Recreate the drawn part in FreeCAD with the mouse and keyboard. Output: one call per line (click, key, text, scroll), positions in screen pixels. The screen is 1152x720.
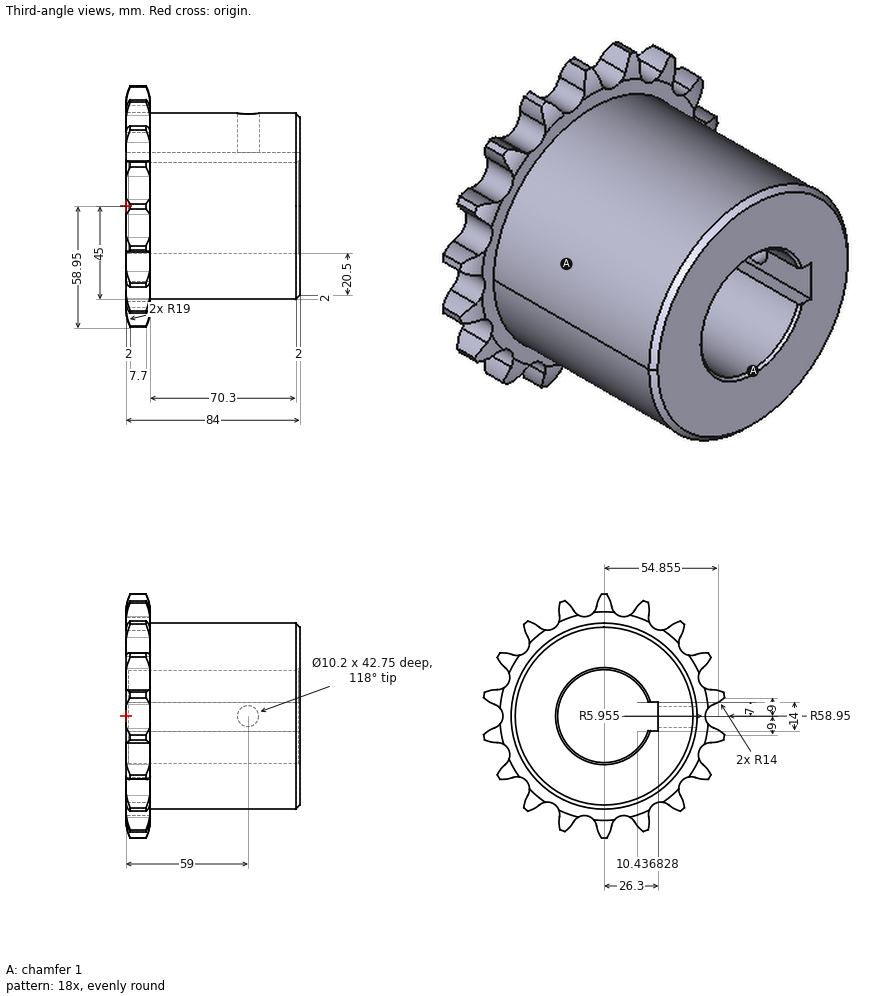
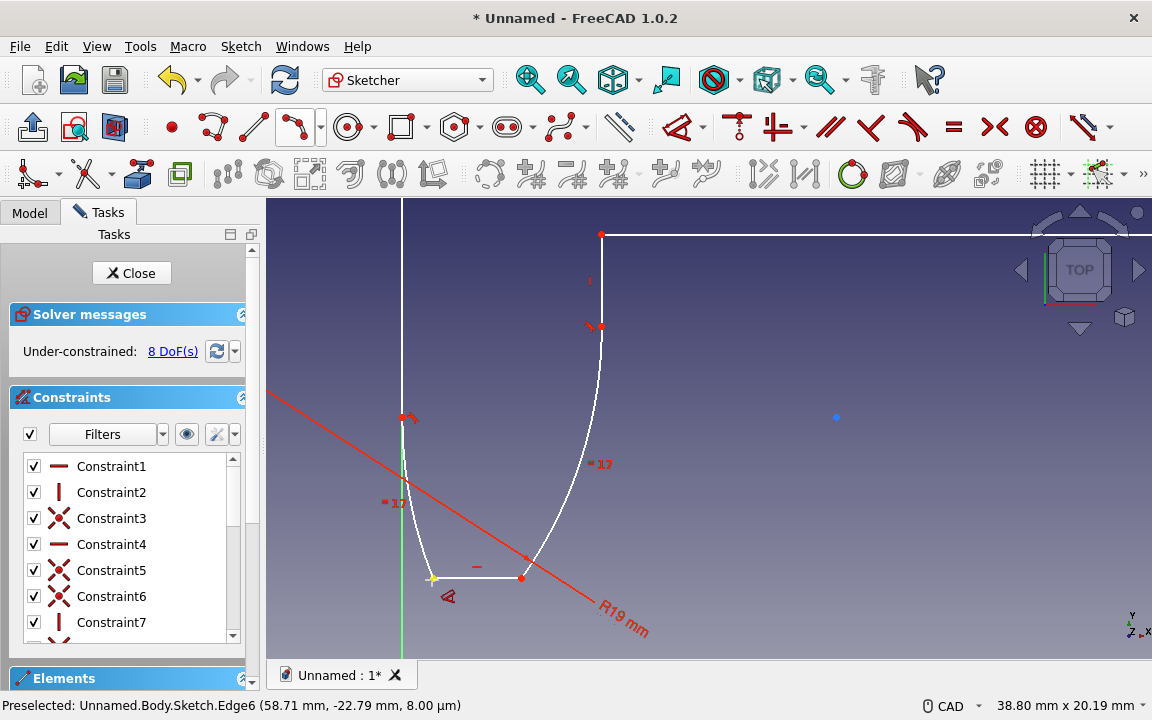
click(433, 578)
click(418, 612)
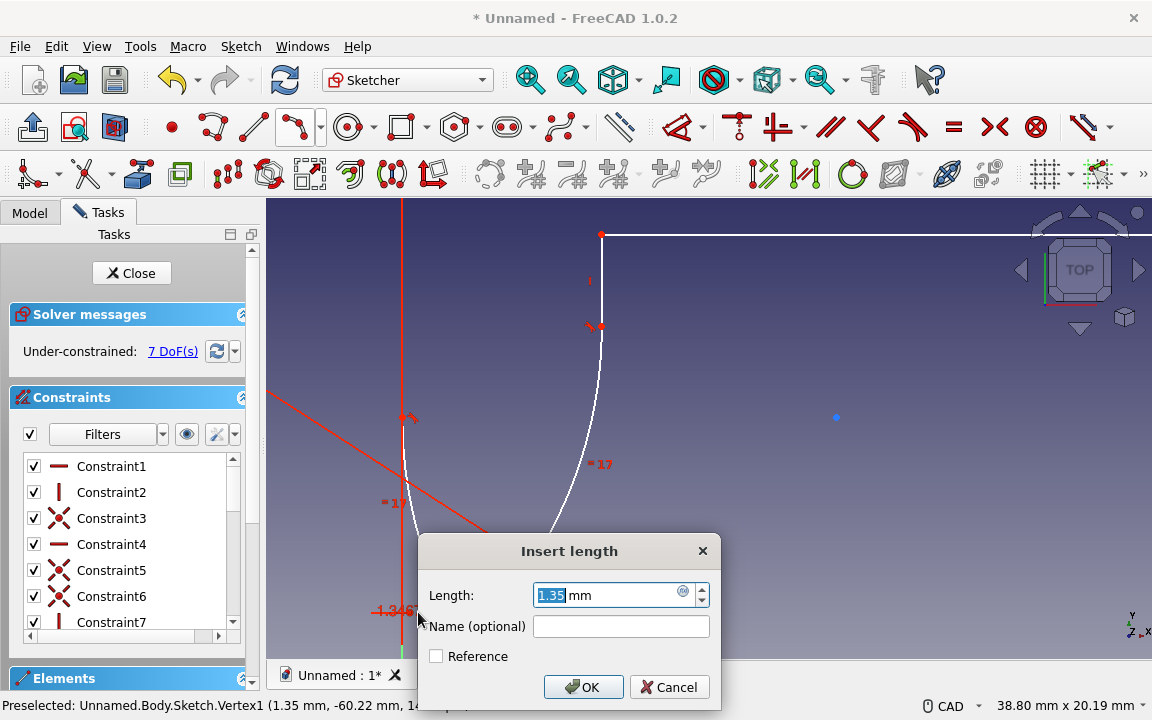
text(2)
key(Return)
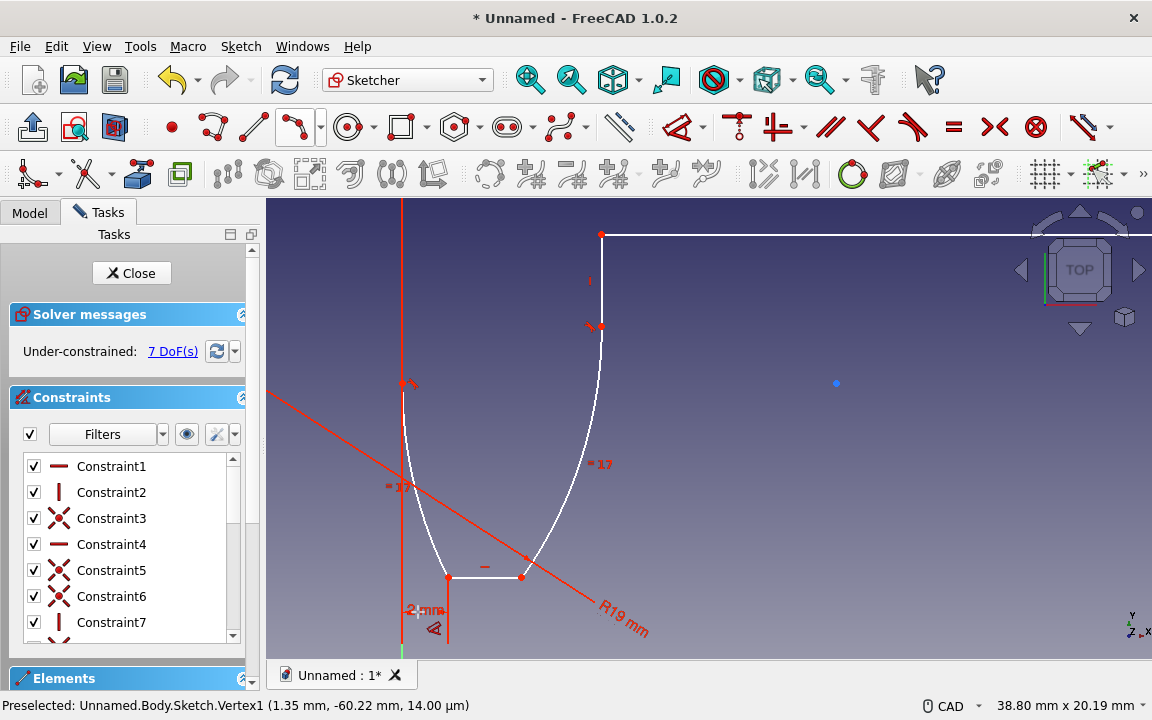
scroll(458, 568, down, 8)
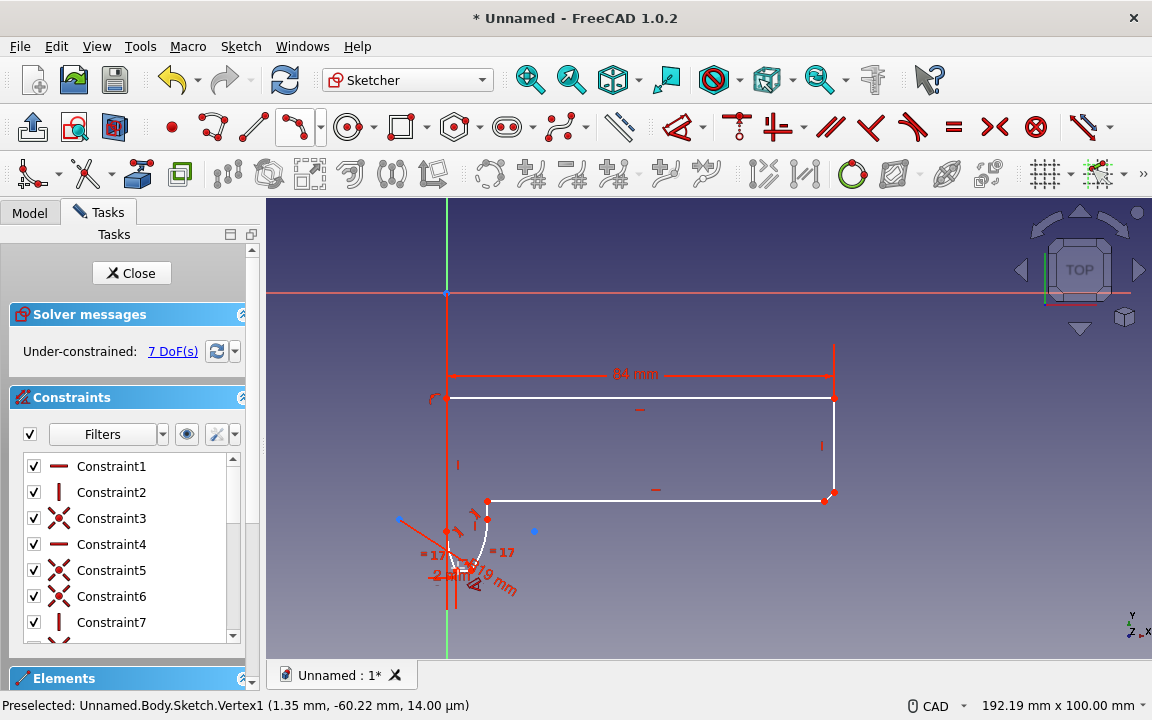
scroll(828, 499, up, 8)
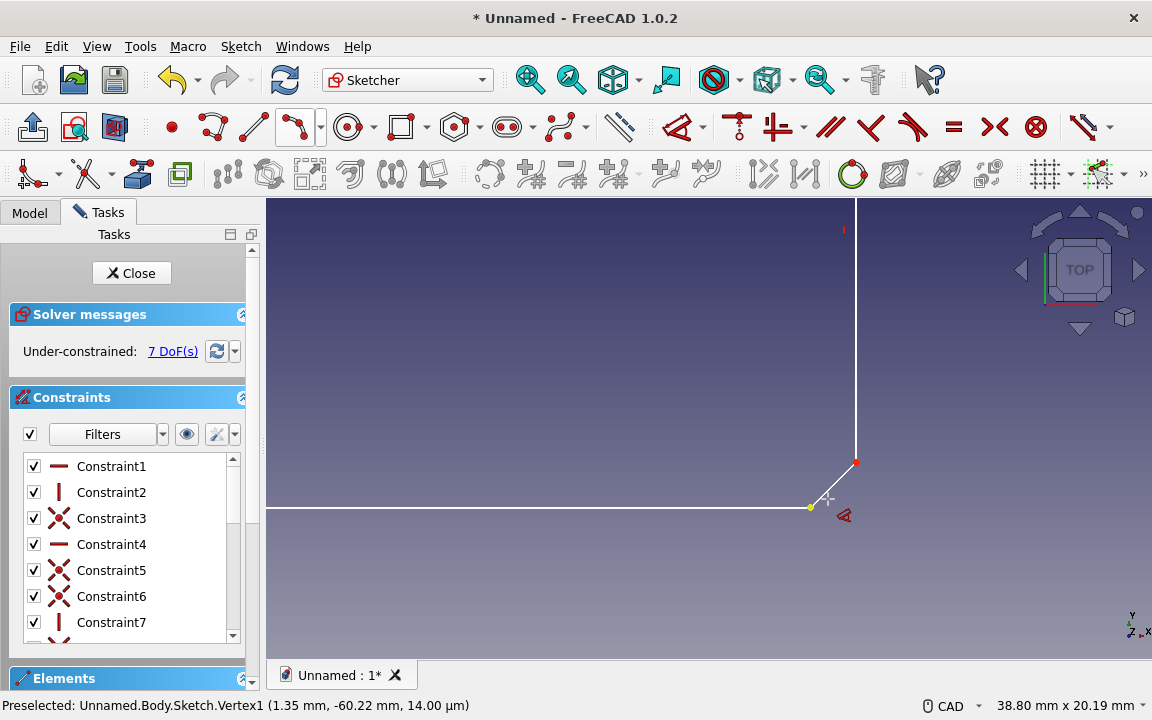
click(824, 494)
click(833, 542)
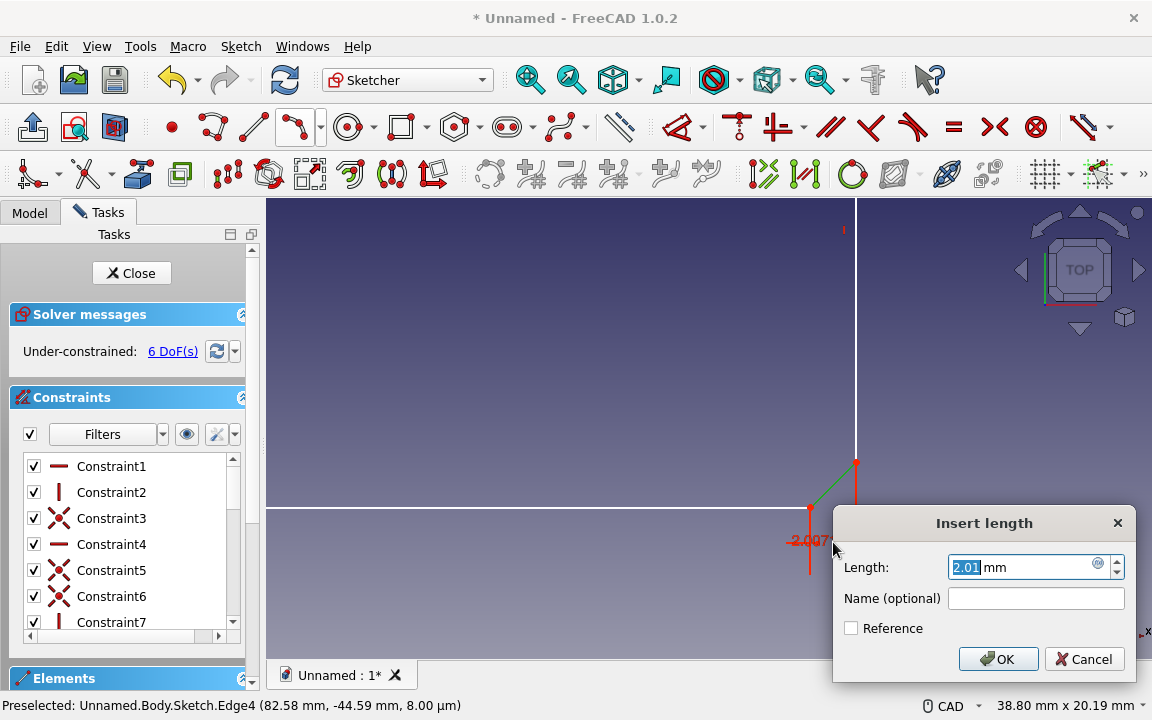
text(2)
key(Return)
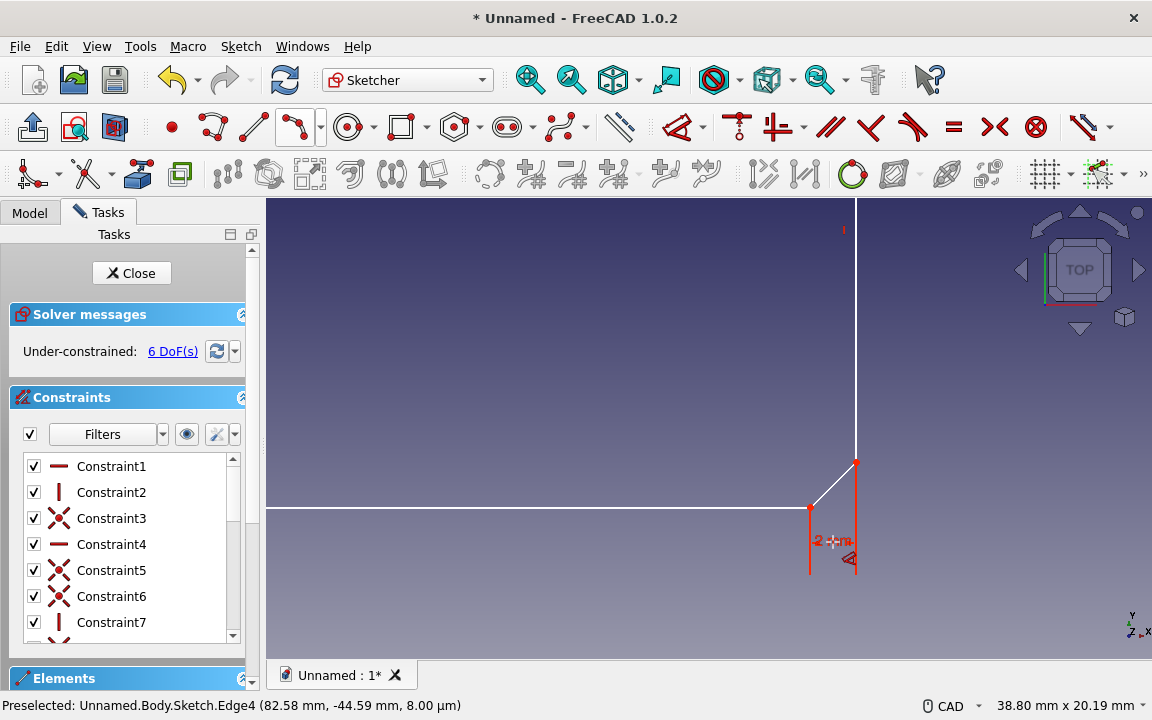
click(824, 494)
click(890, 485)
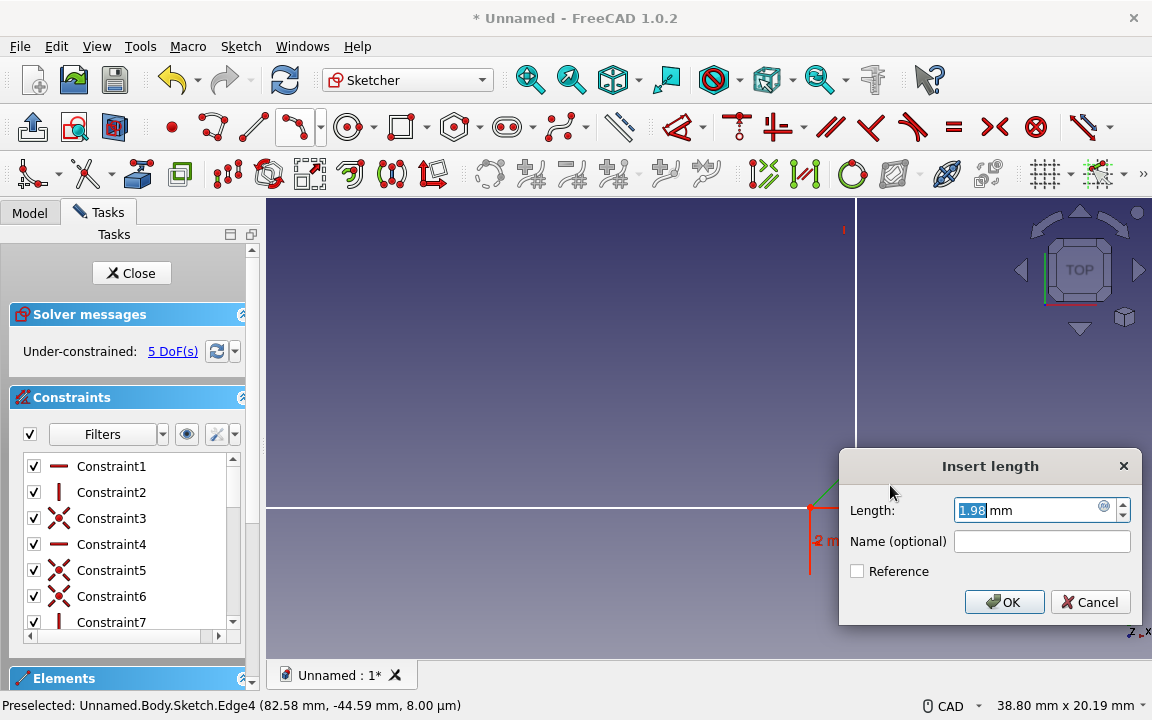
text(2)
key(Return)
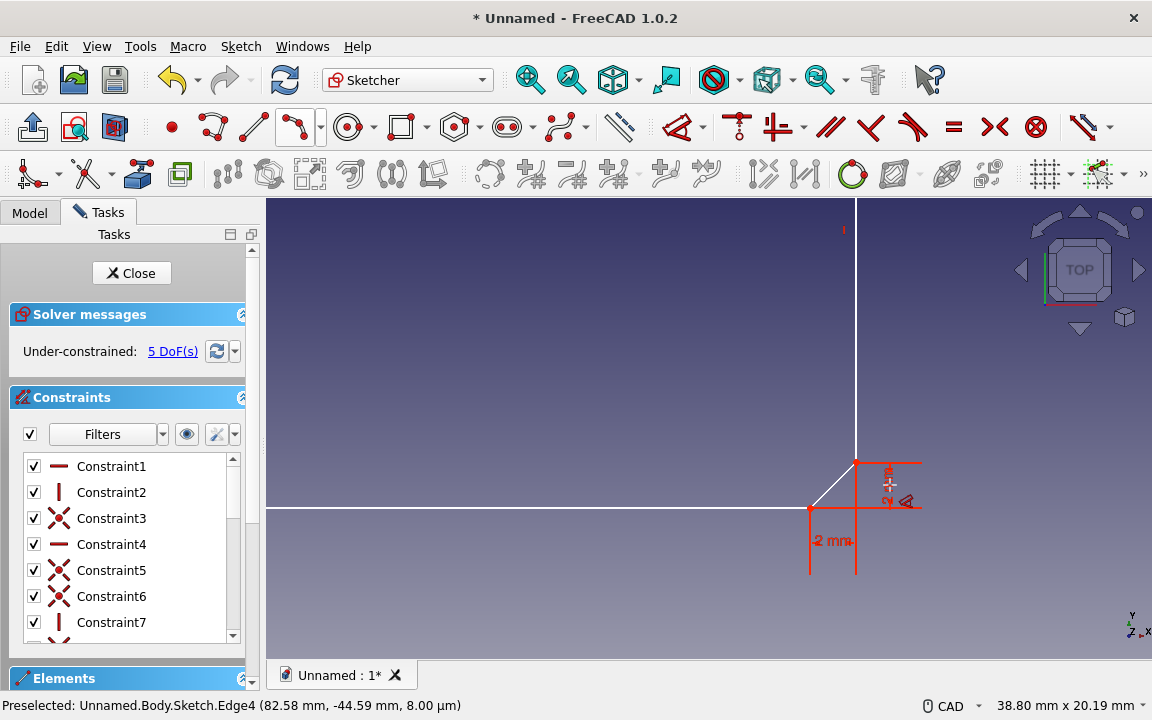
scroll(829, 499, down, 8)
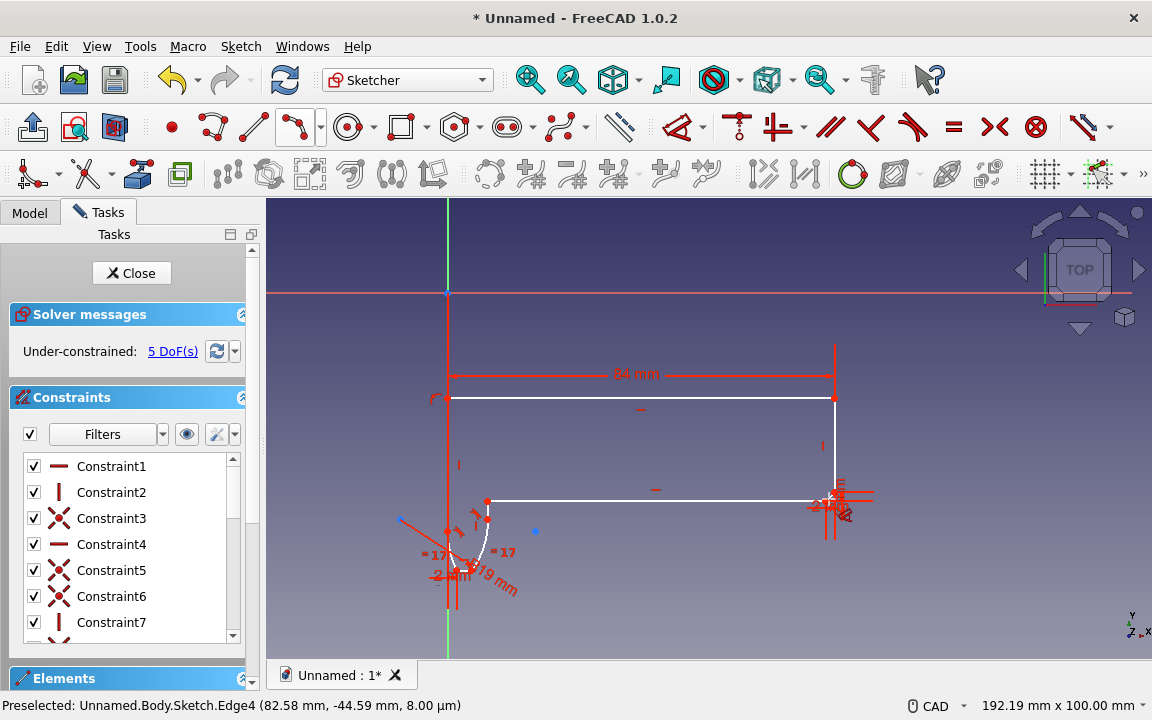
scroll(461, 571, up, 6)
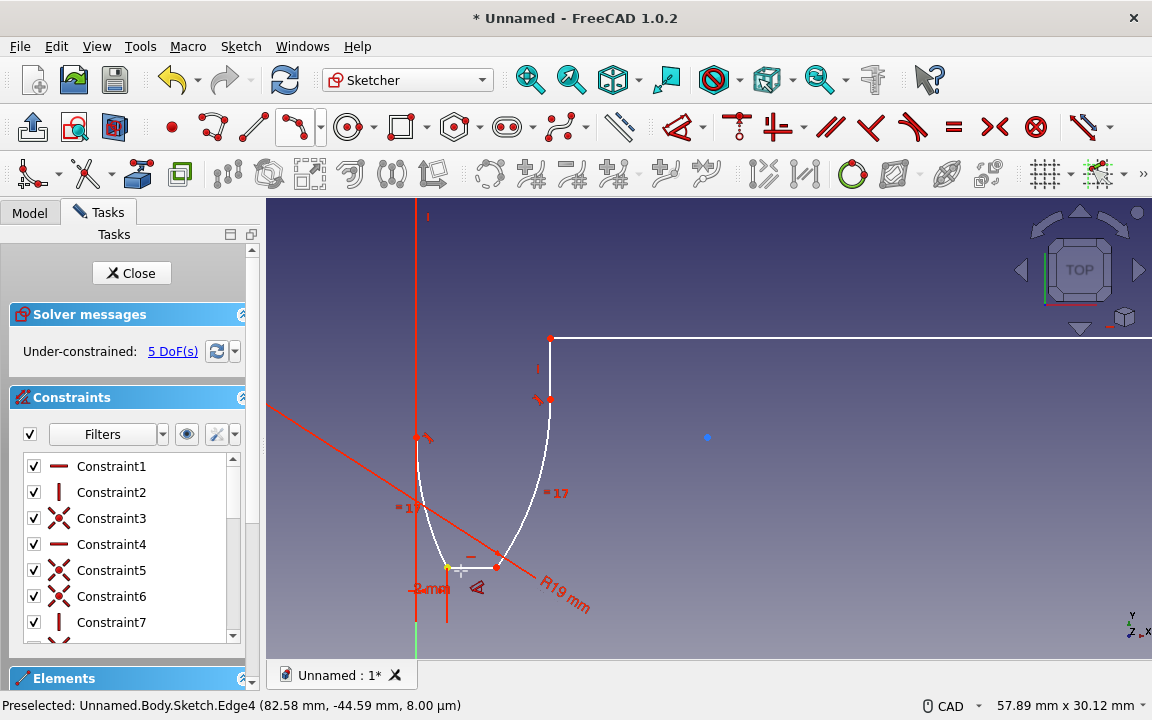
click(462, 568)
click(460, 534)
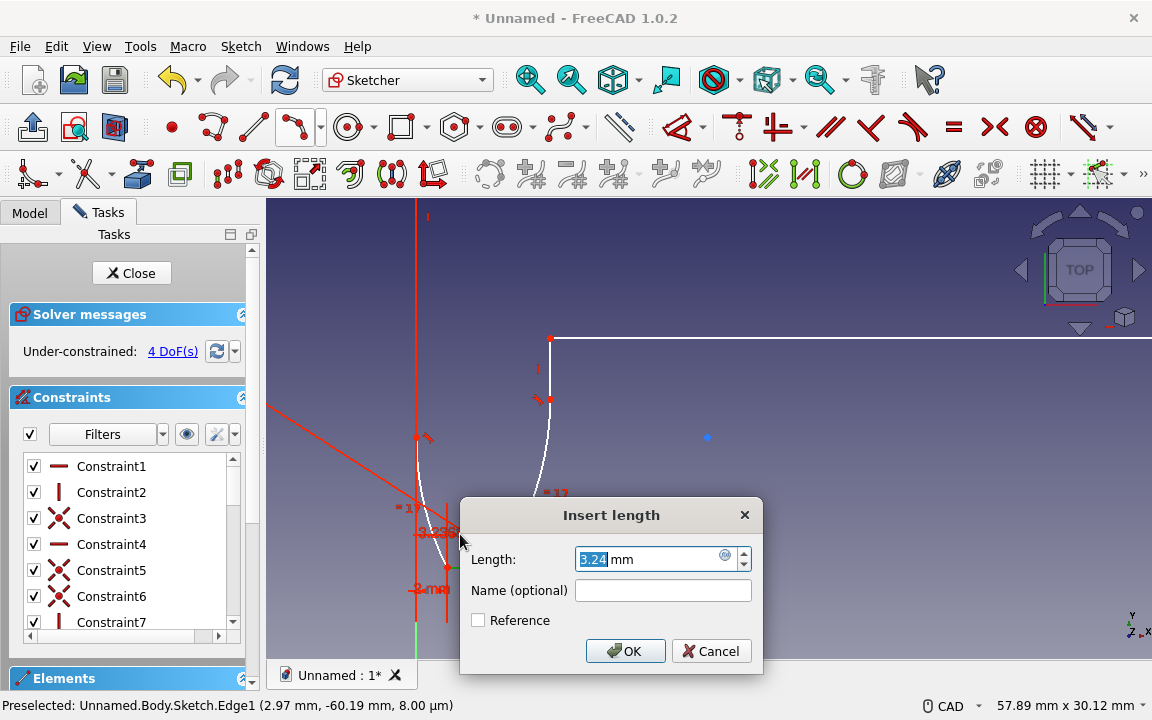
text(7.7)
key(Return)